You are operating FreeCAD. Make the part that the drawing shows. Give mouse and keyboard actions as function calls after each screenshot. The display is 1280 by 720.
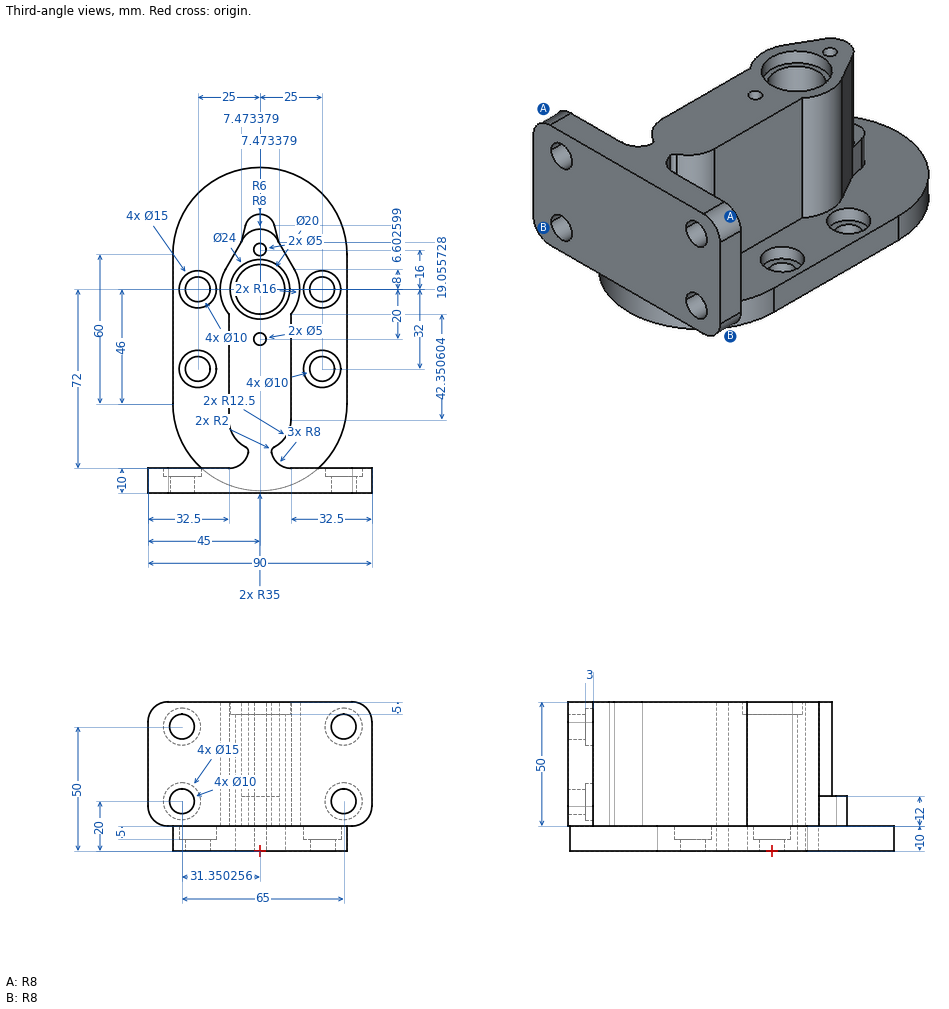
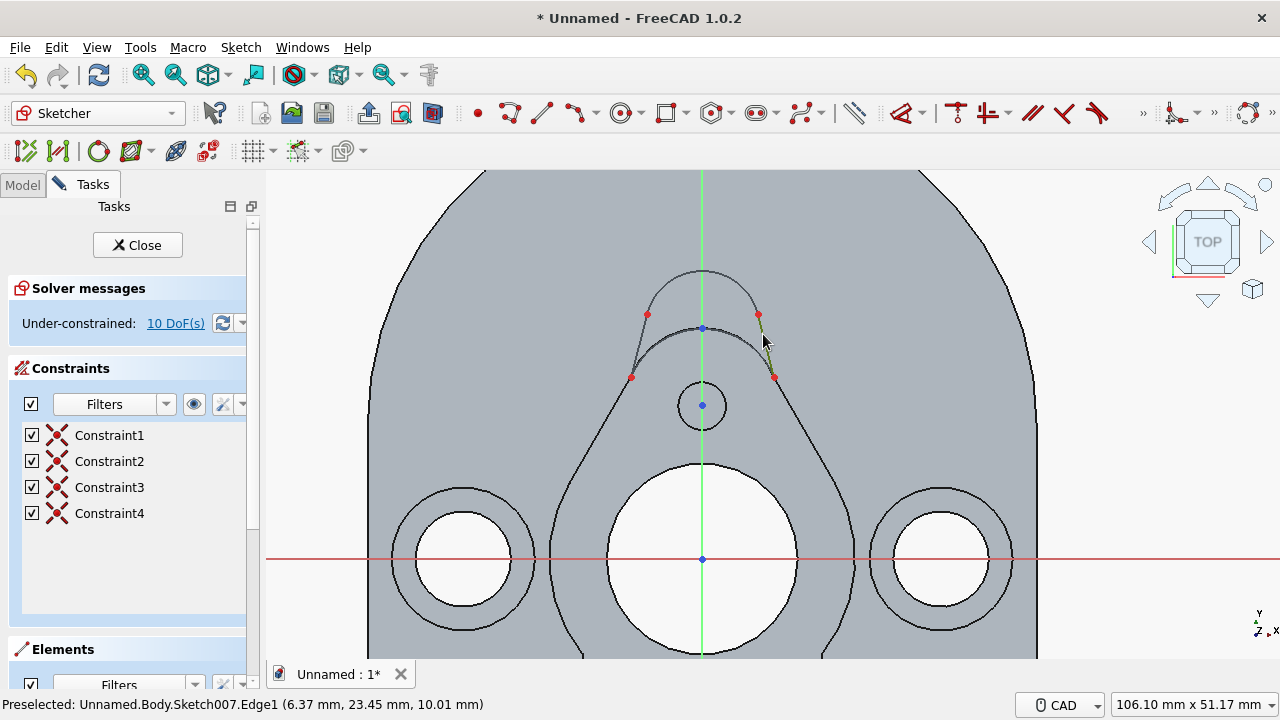
click(732, 279)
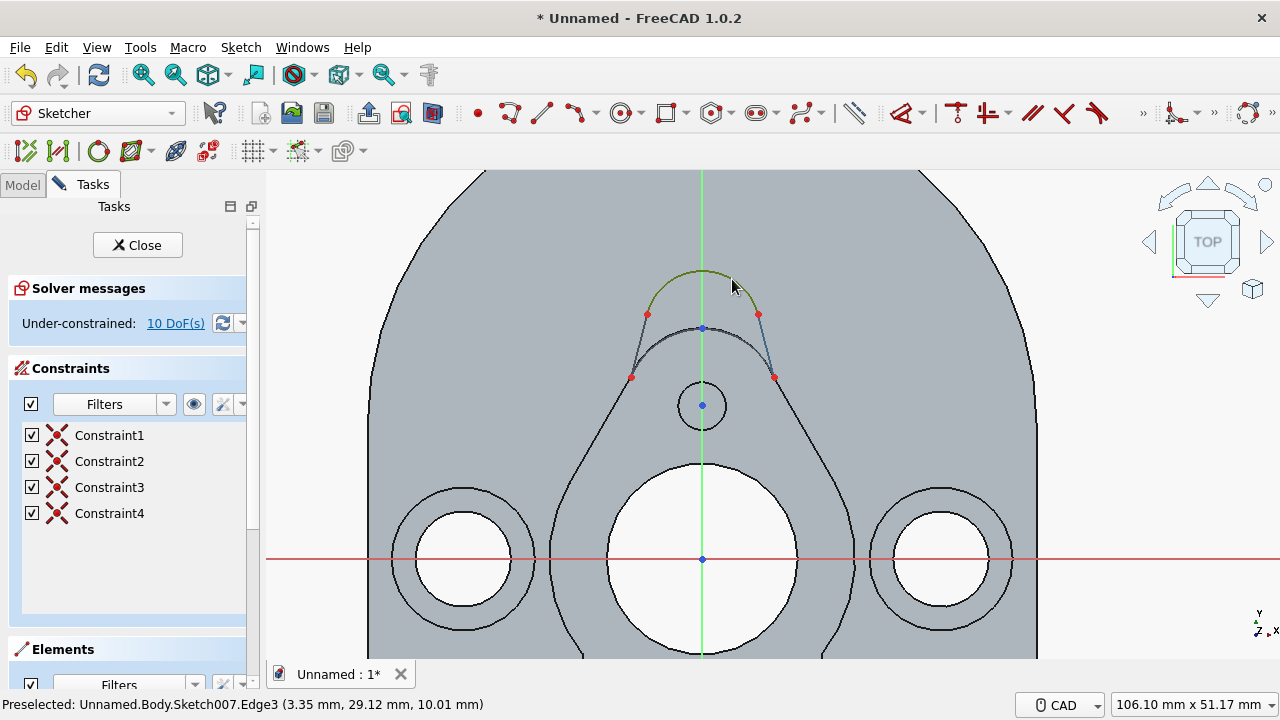
click(1098, 114)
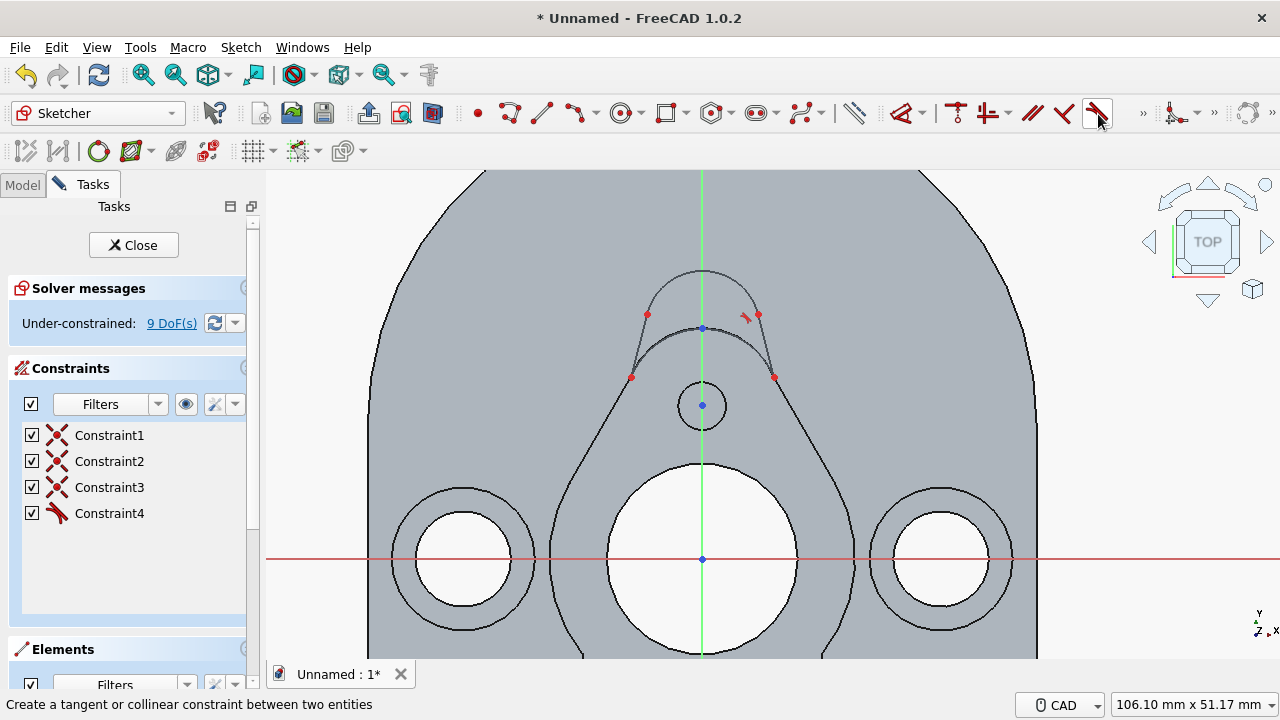
click(642, 334)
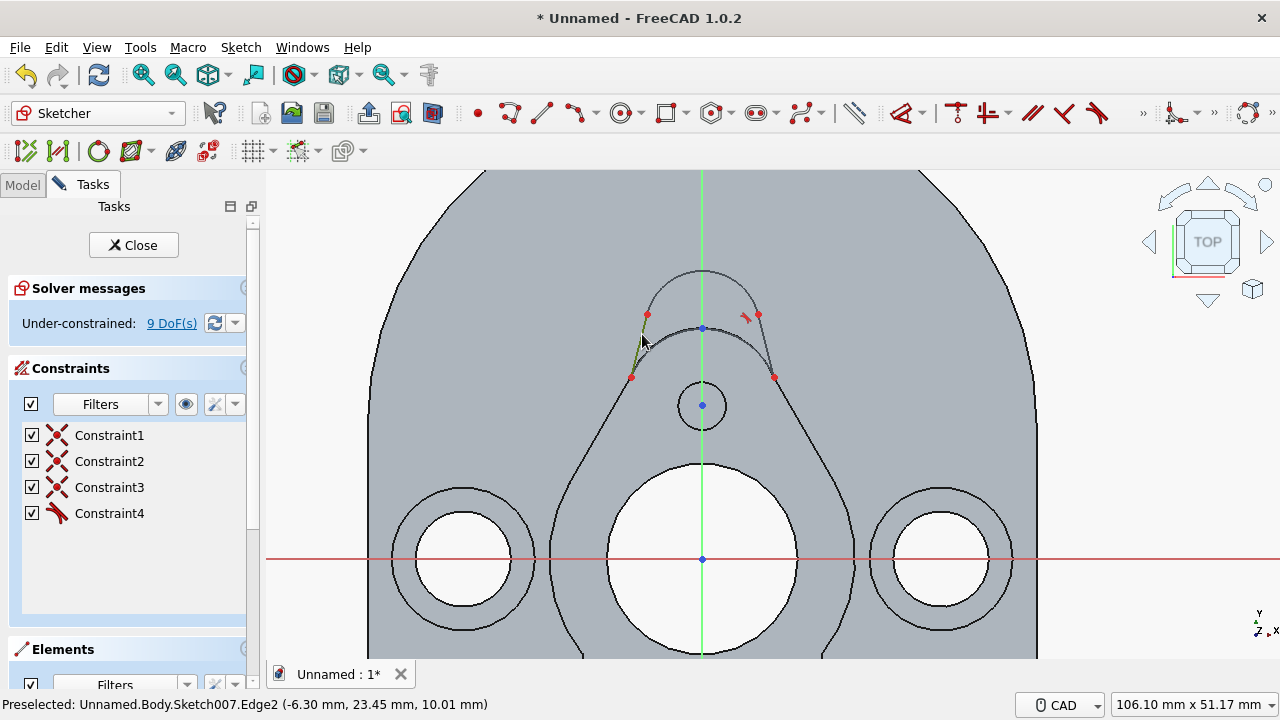
click(731, 279)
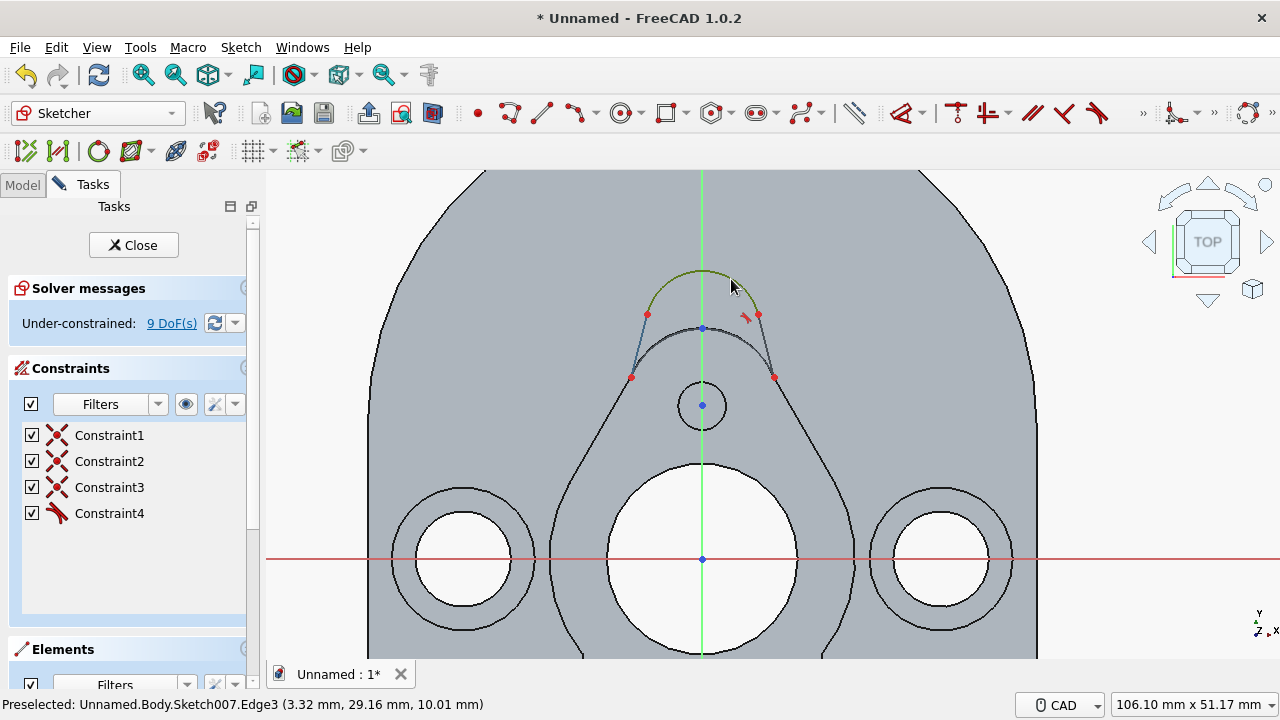
click(1098, 114)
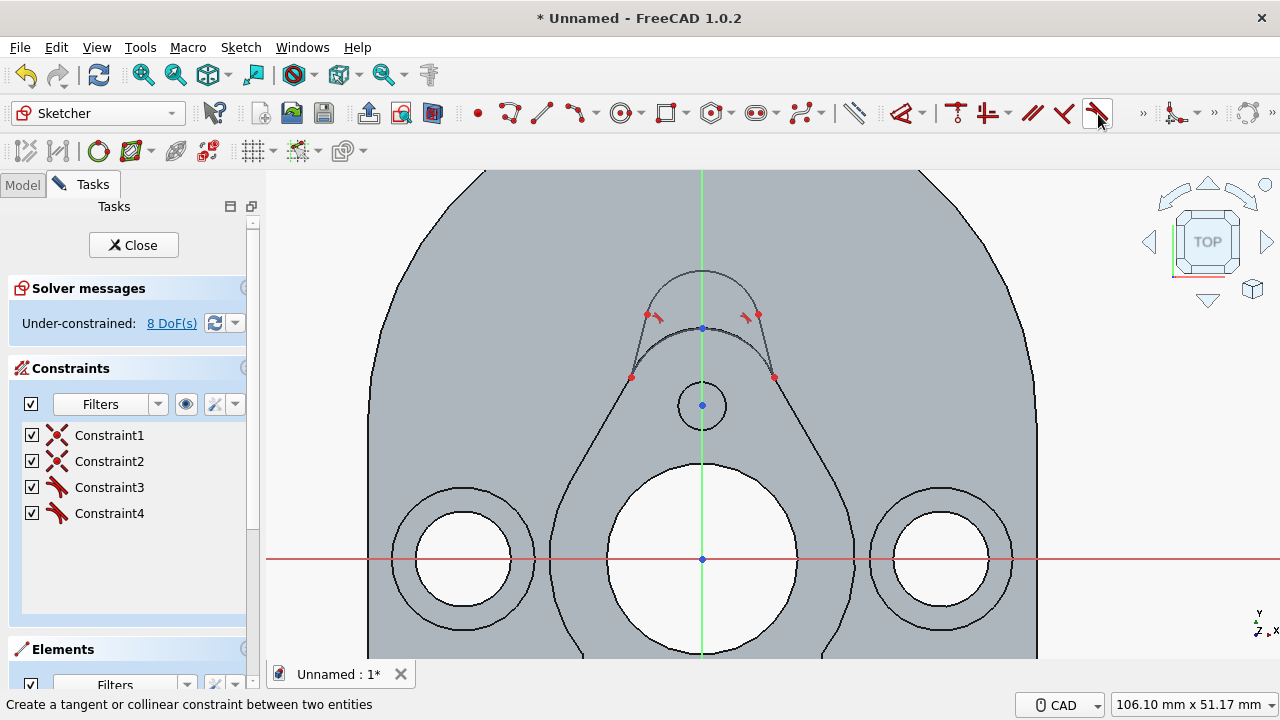
click(703, 328)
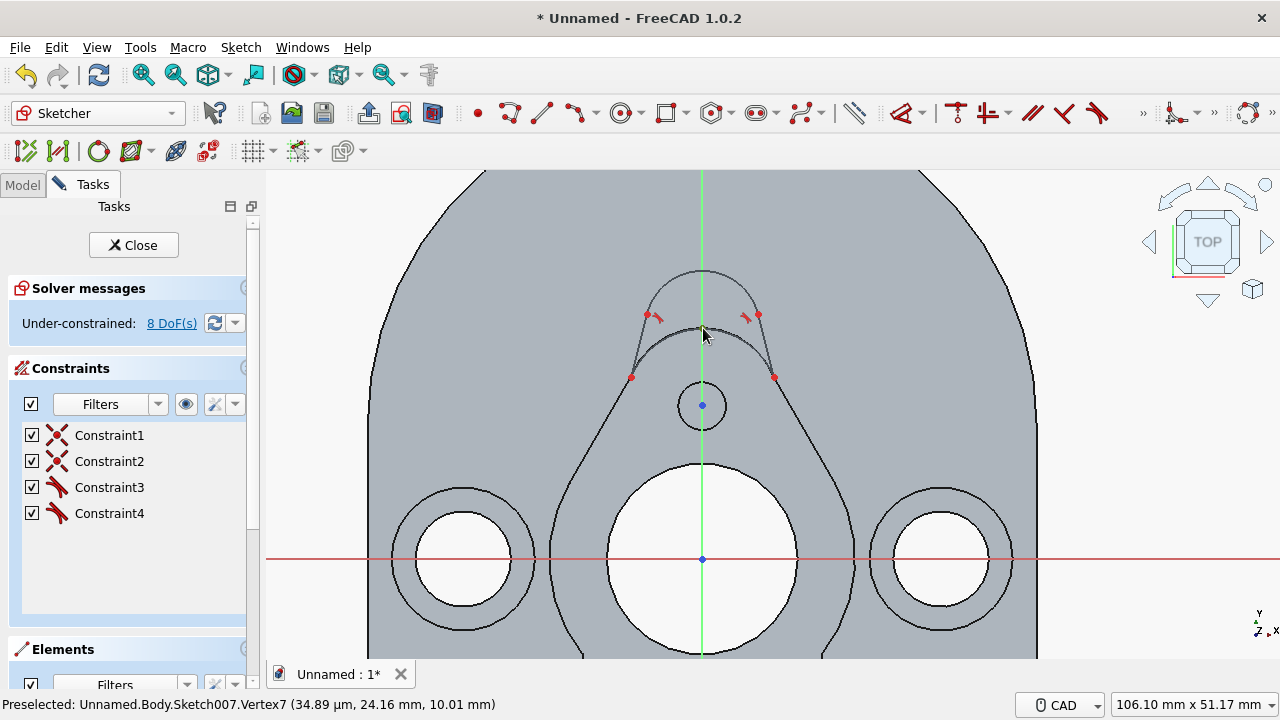
click(702, 600)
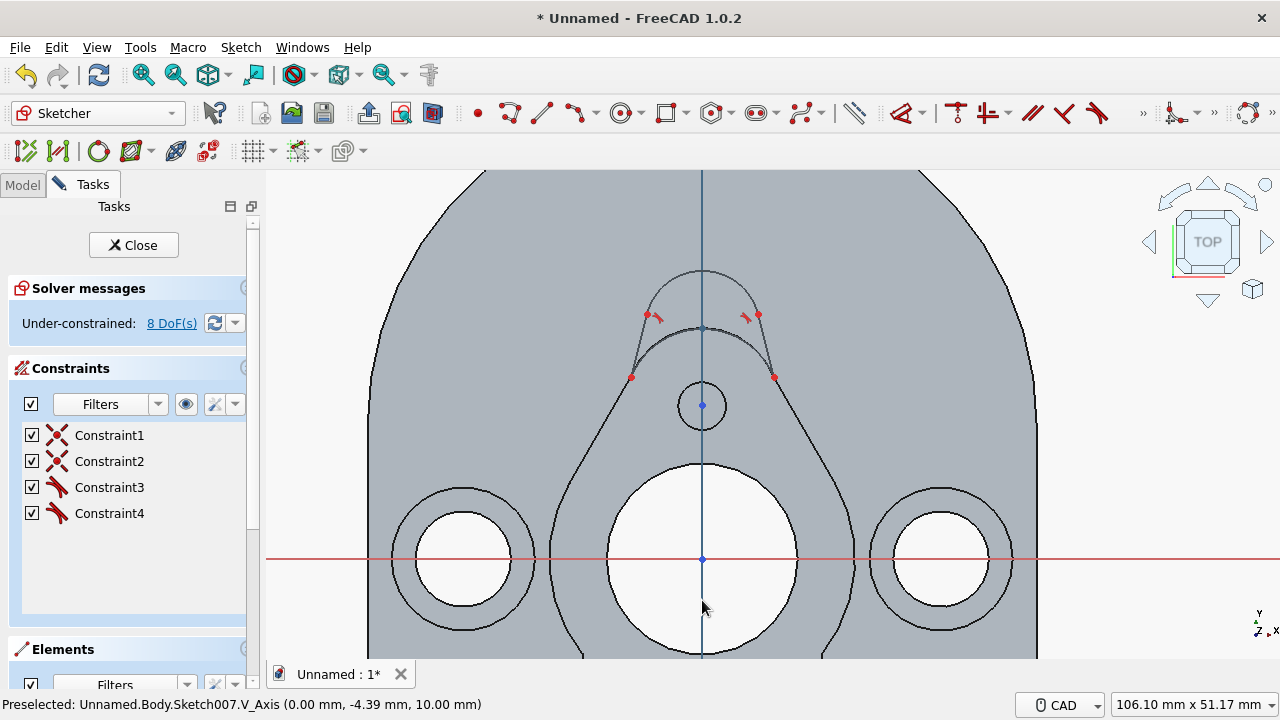
click(956, 114)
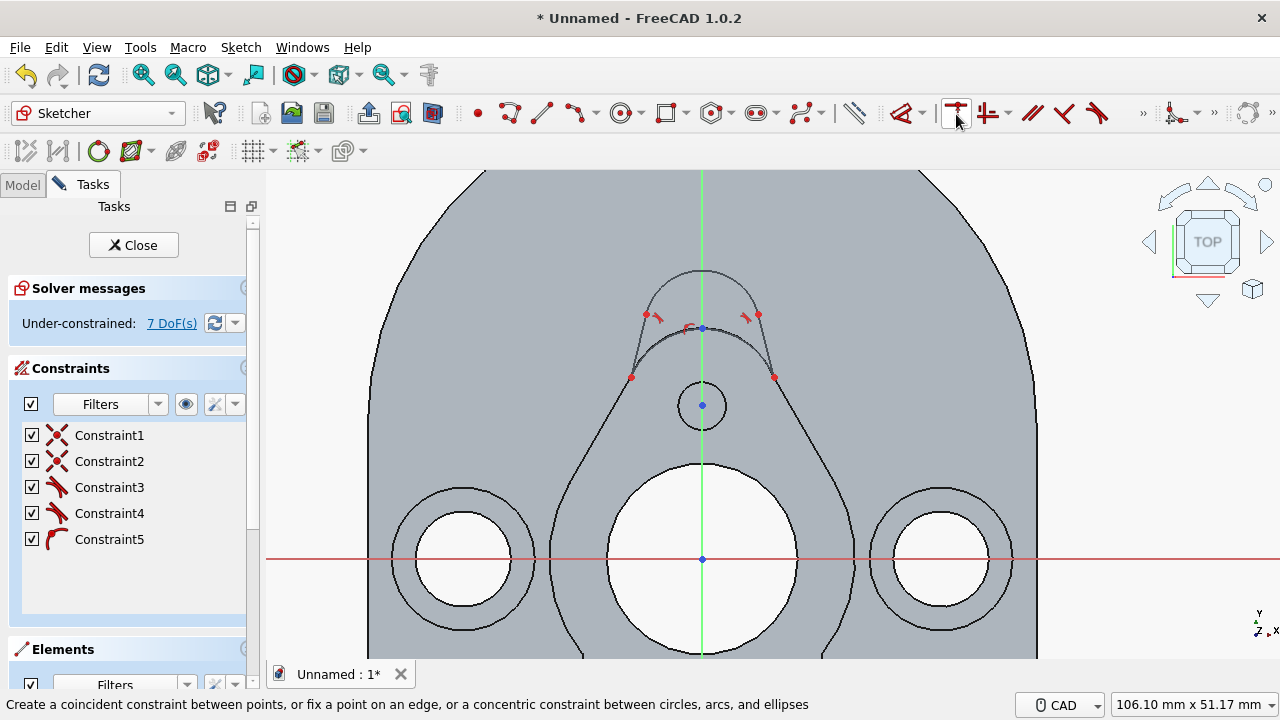
click(703, 406)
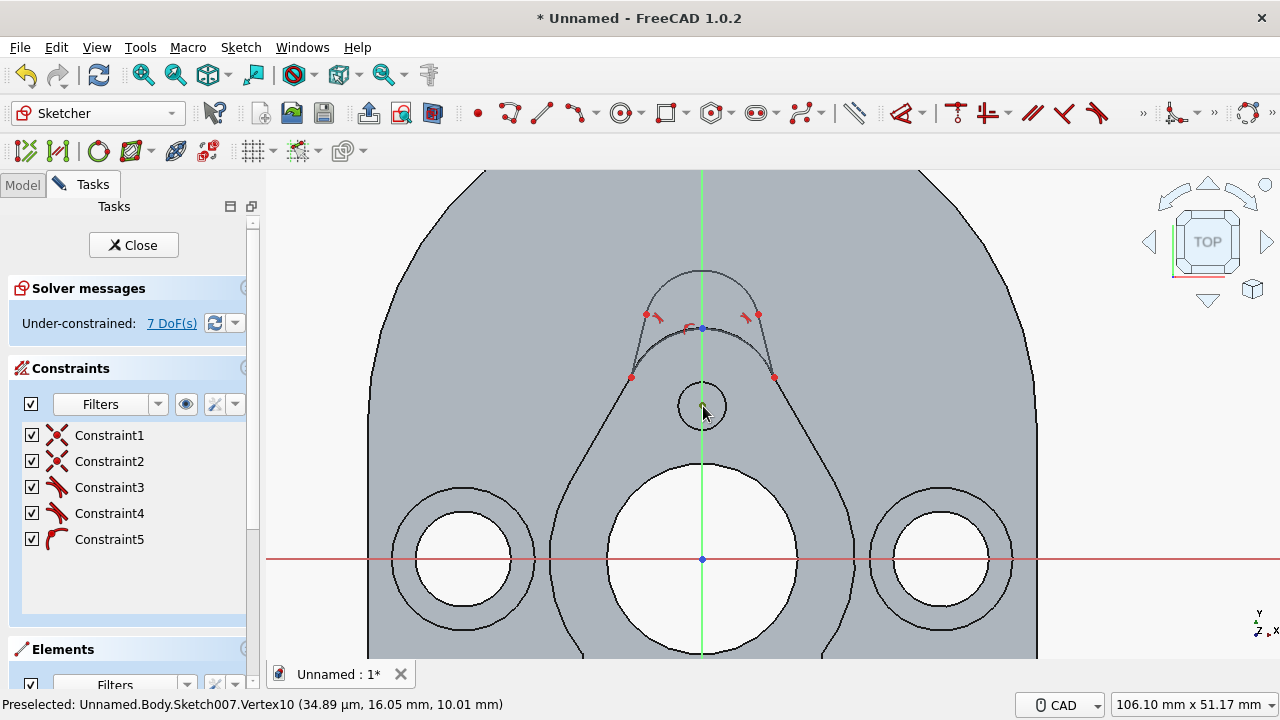
click(702, 600)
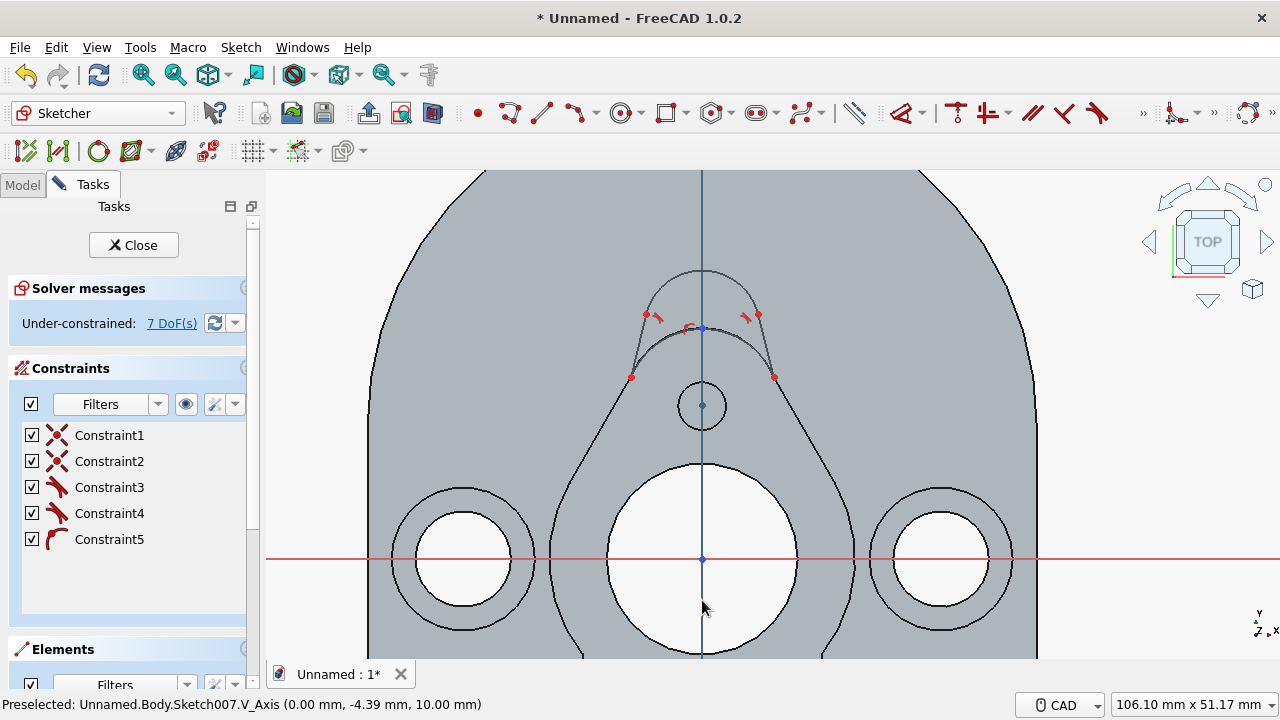
click(956, 114)